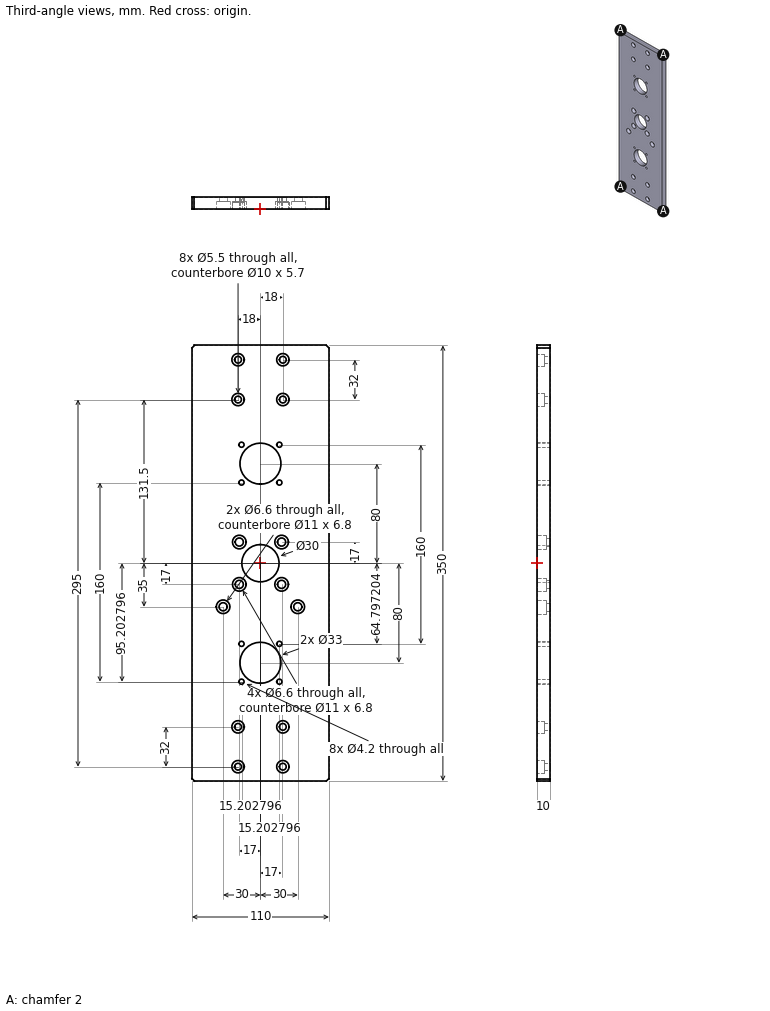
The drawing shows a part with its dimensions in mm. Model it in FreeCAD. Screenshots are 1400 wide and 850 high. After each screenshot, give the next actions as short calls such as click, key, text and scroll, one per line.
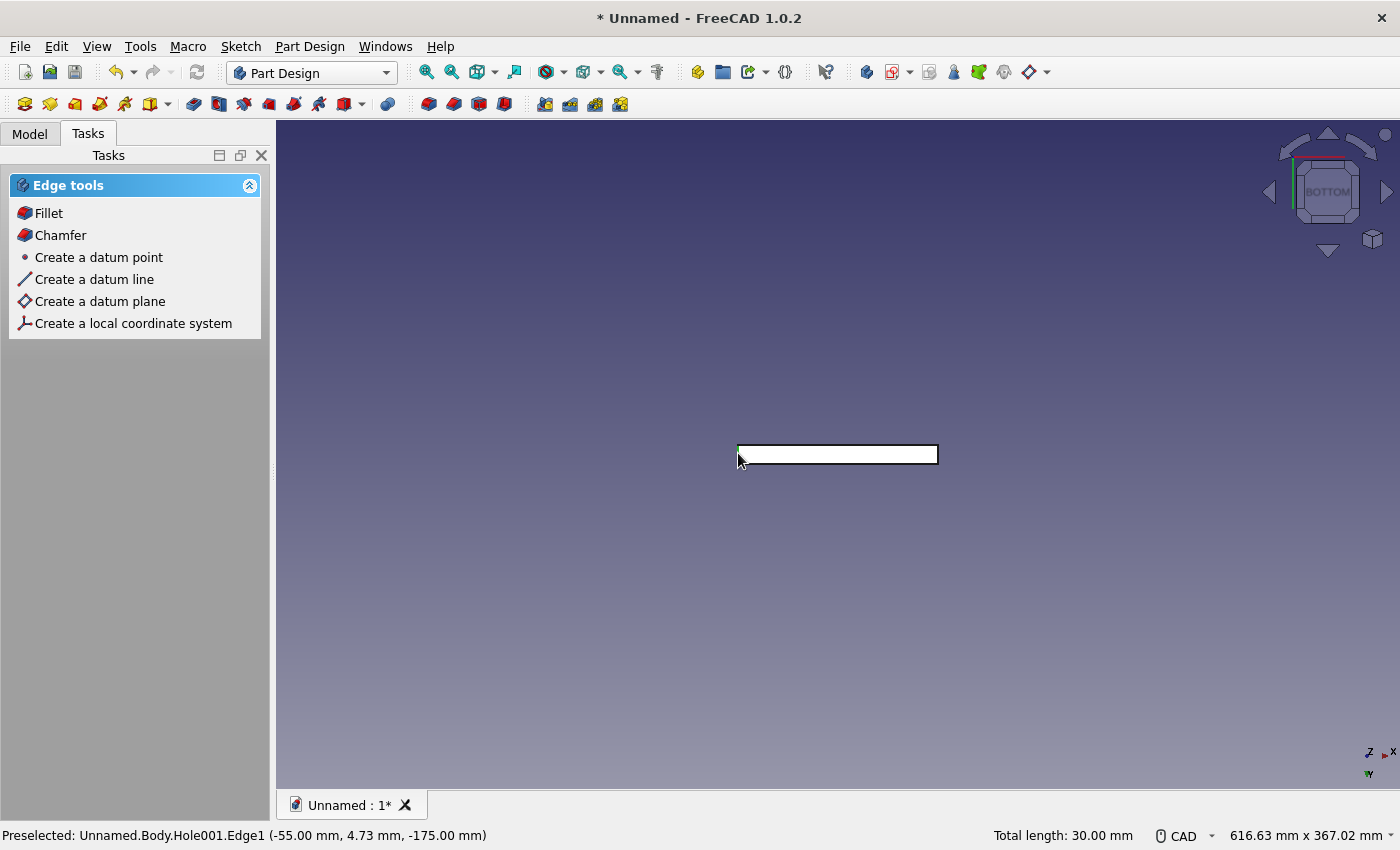
click(938, 453, ctrl)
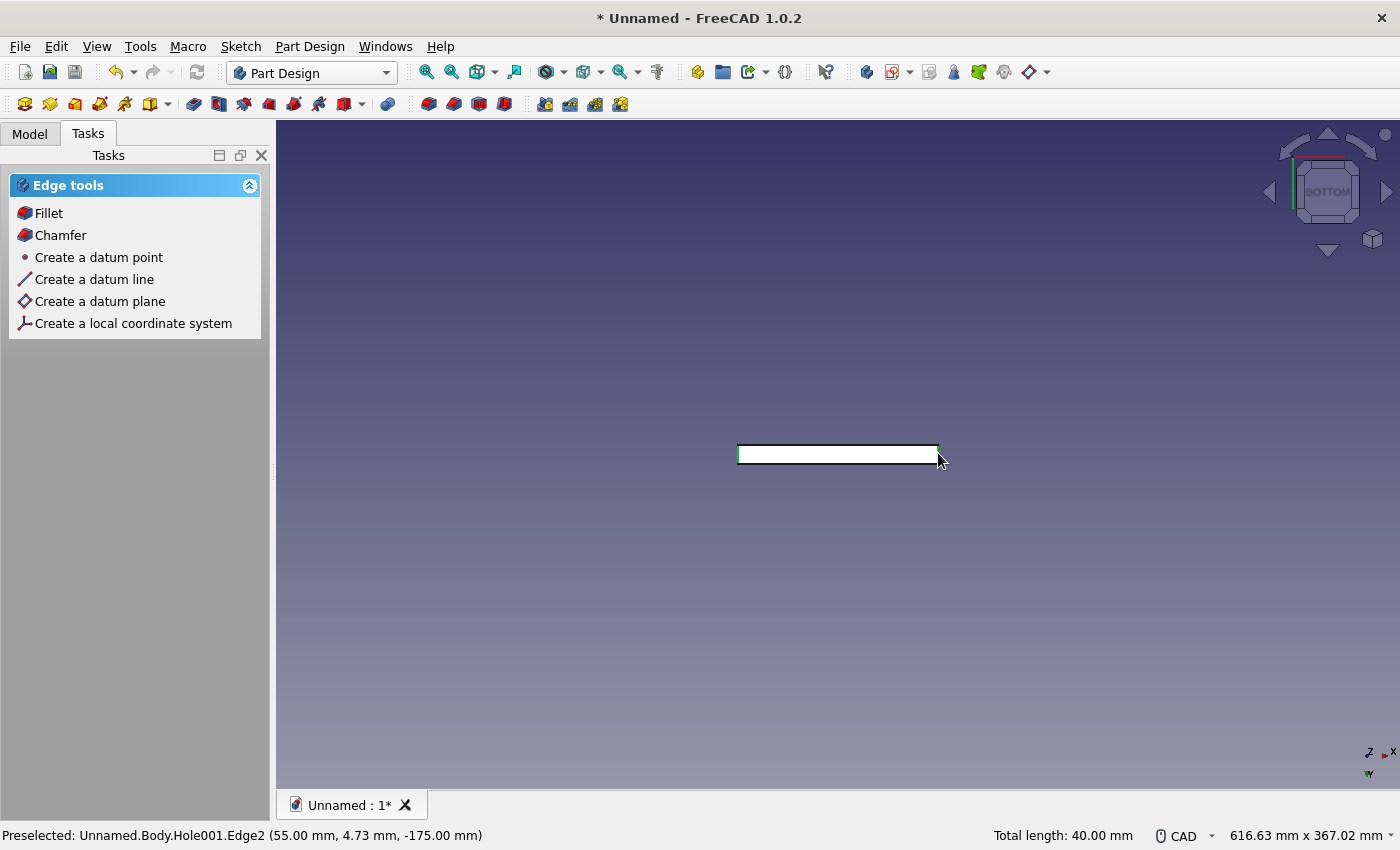
click(454, 104)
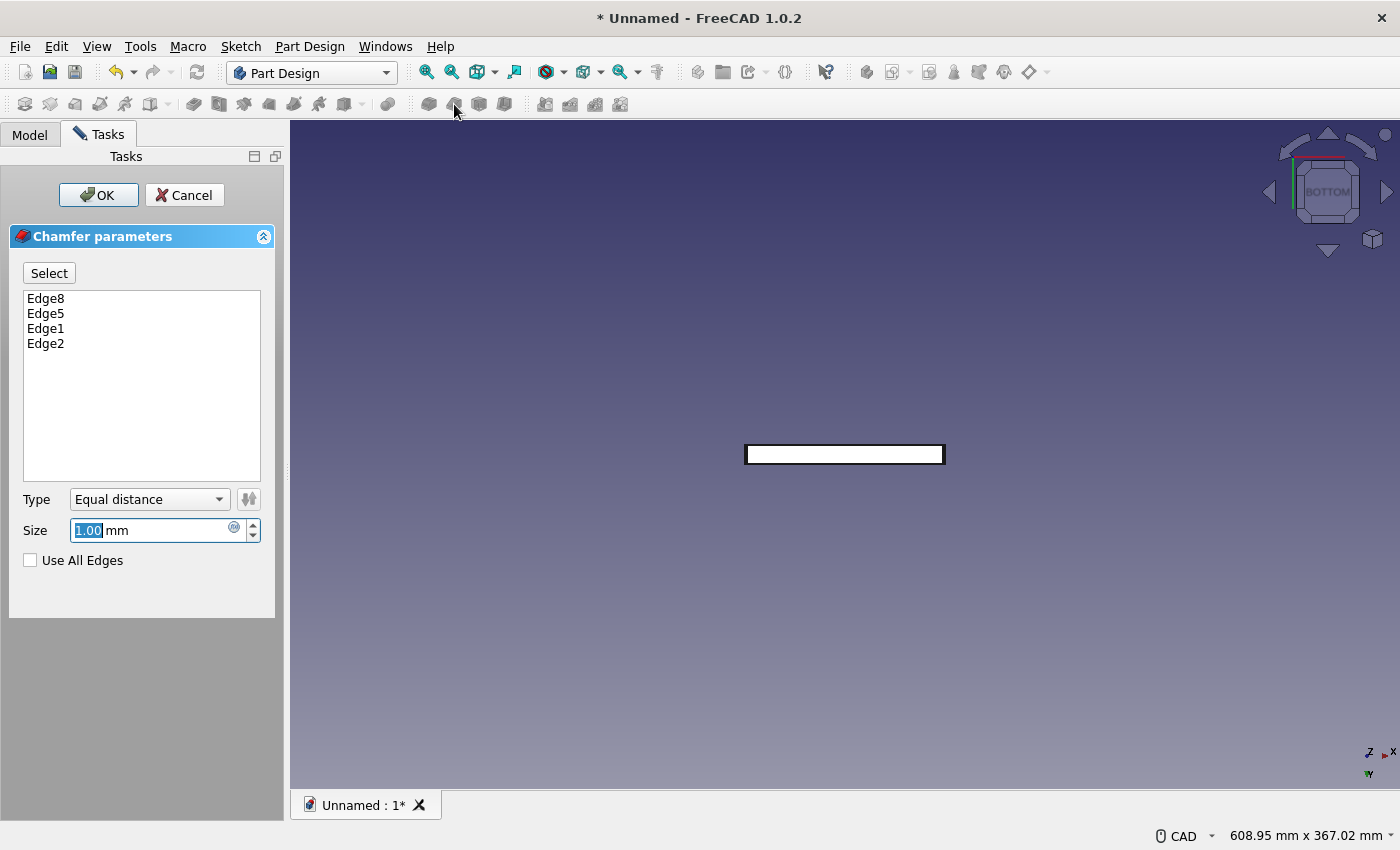
text(2)
key(Tab)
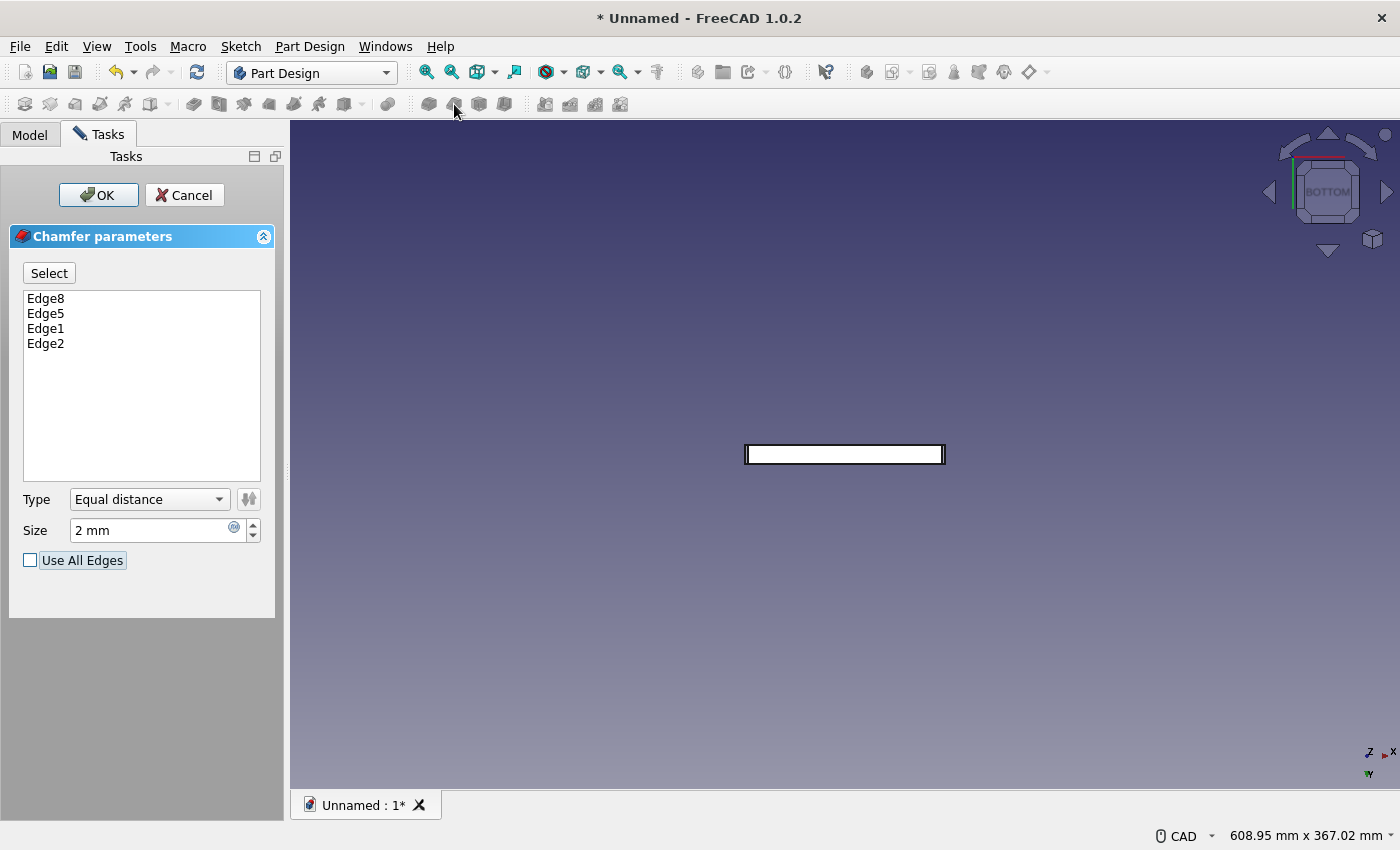
click(99, 195)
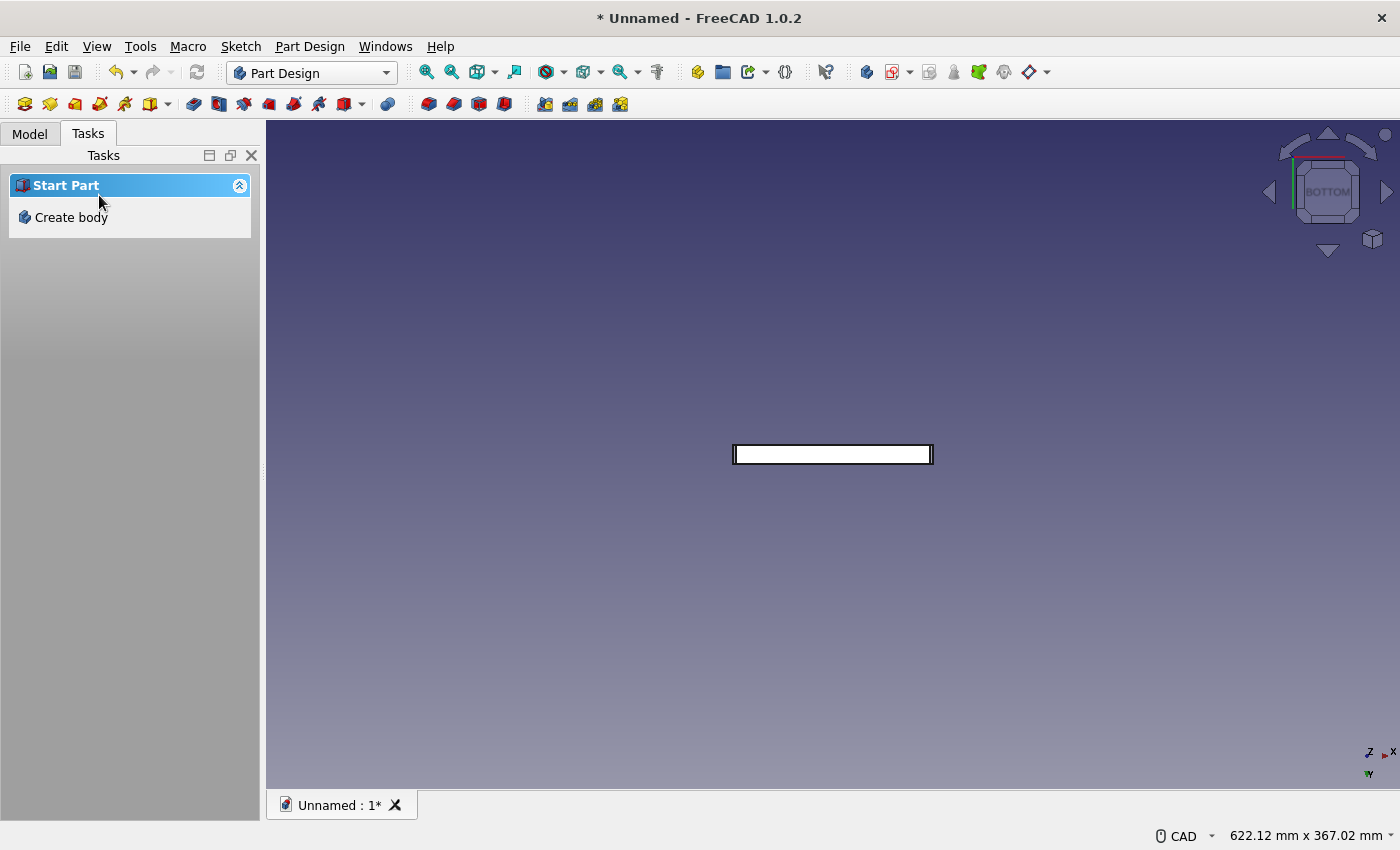
click(427, 72)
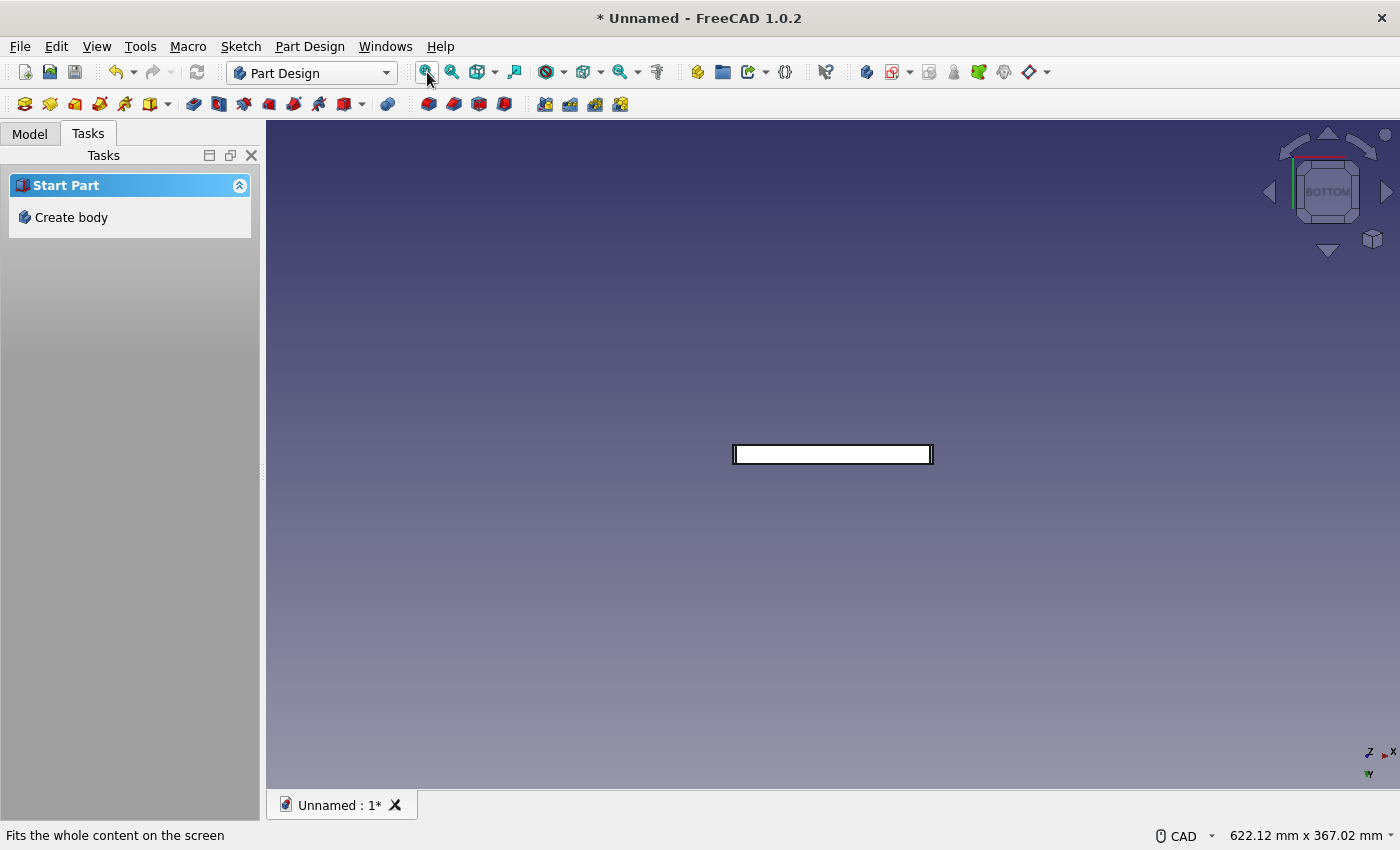
key(0)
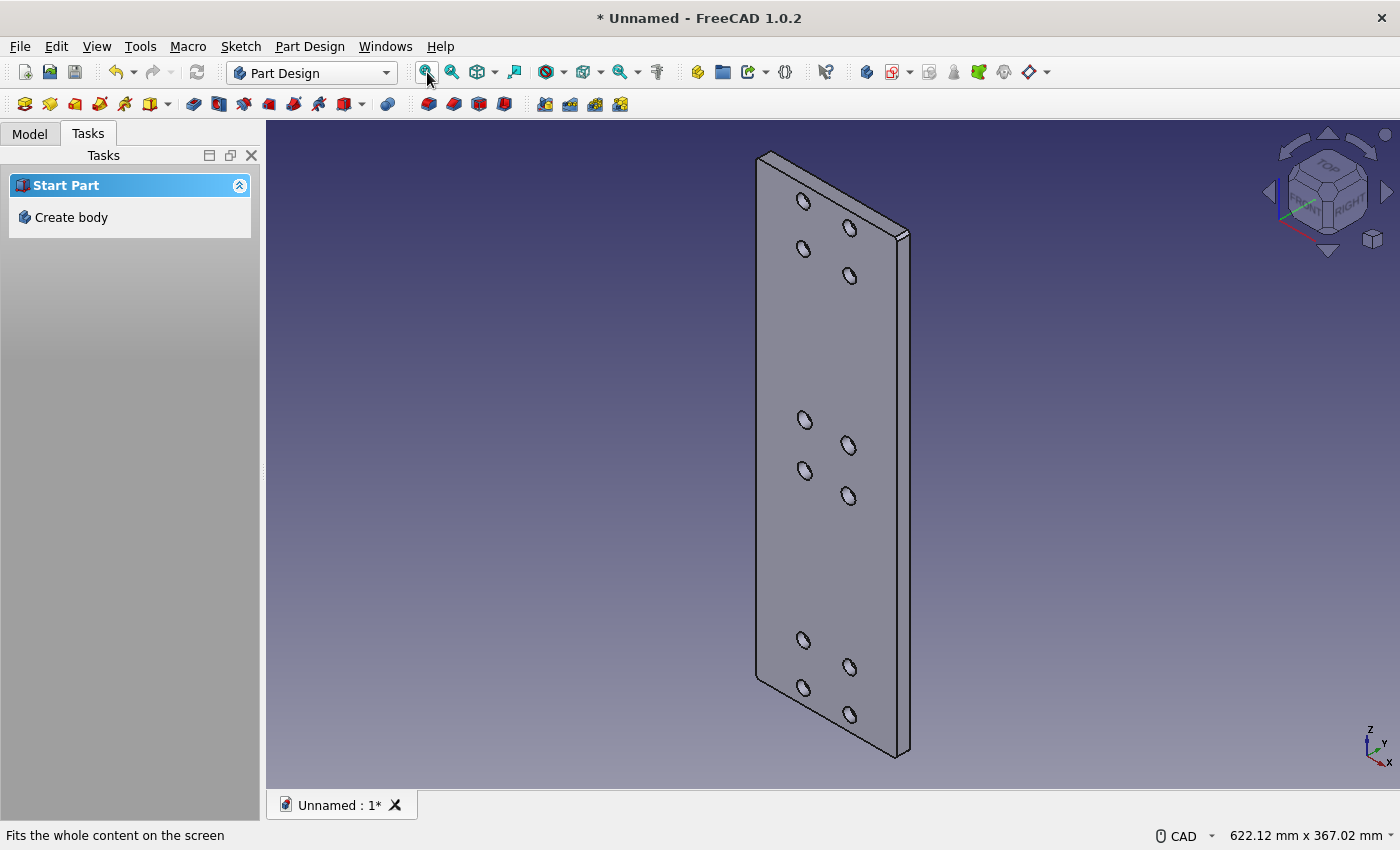
click(827, 383)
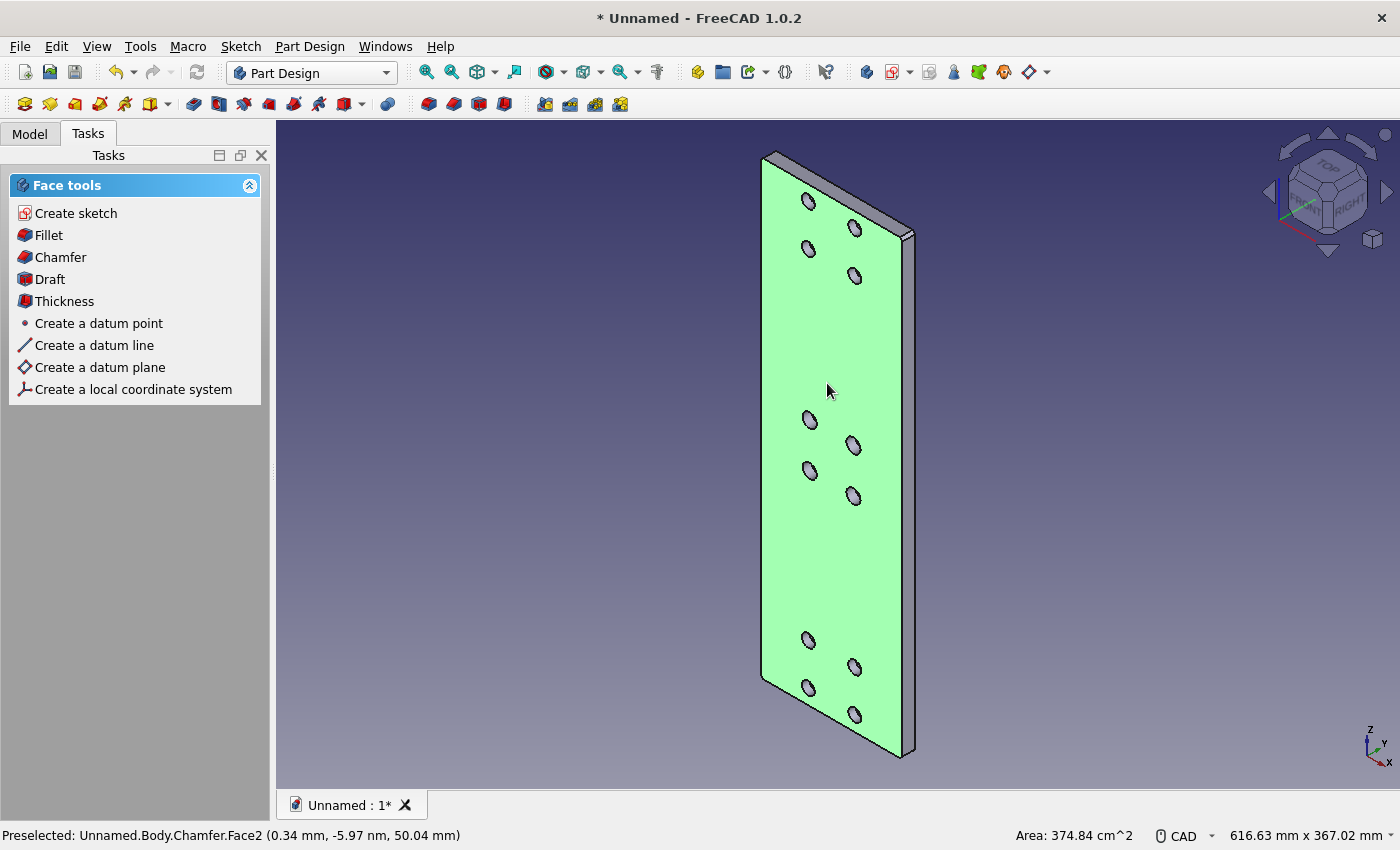
click(892, 72)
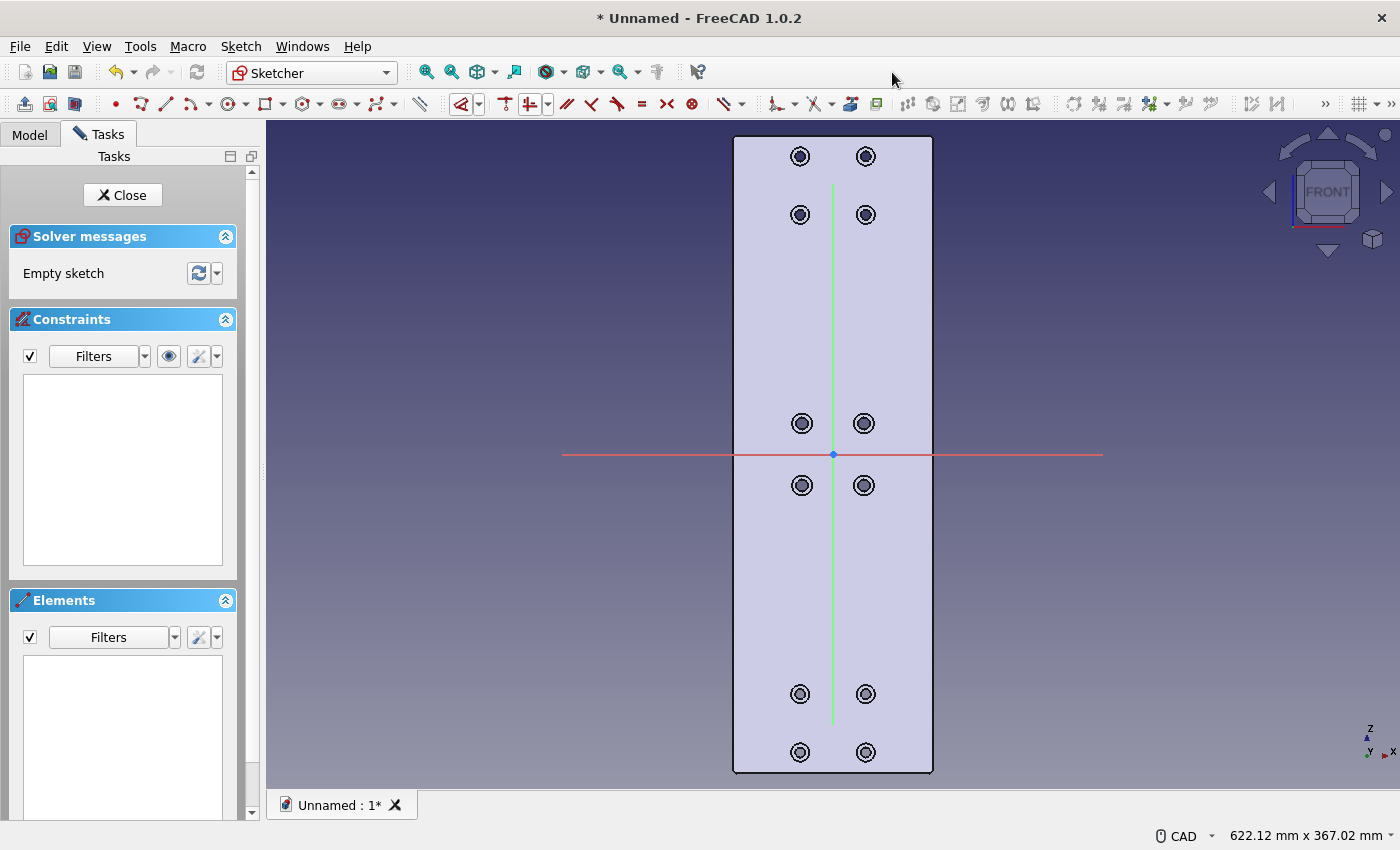
scroll(850, 498, up, 8)